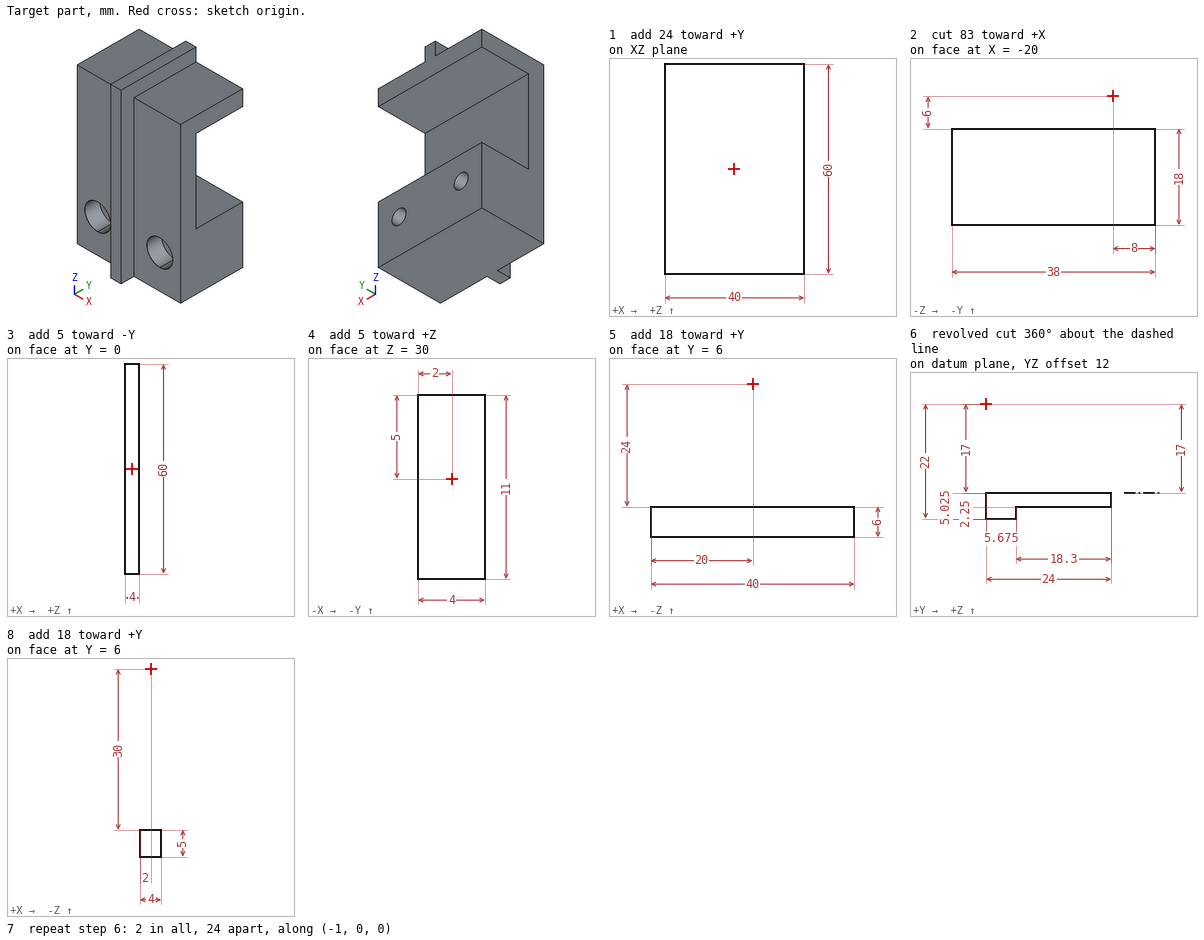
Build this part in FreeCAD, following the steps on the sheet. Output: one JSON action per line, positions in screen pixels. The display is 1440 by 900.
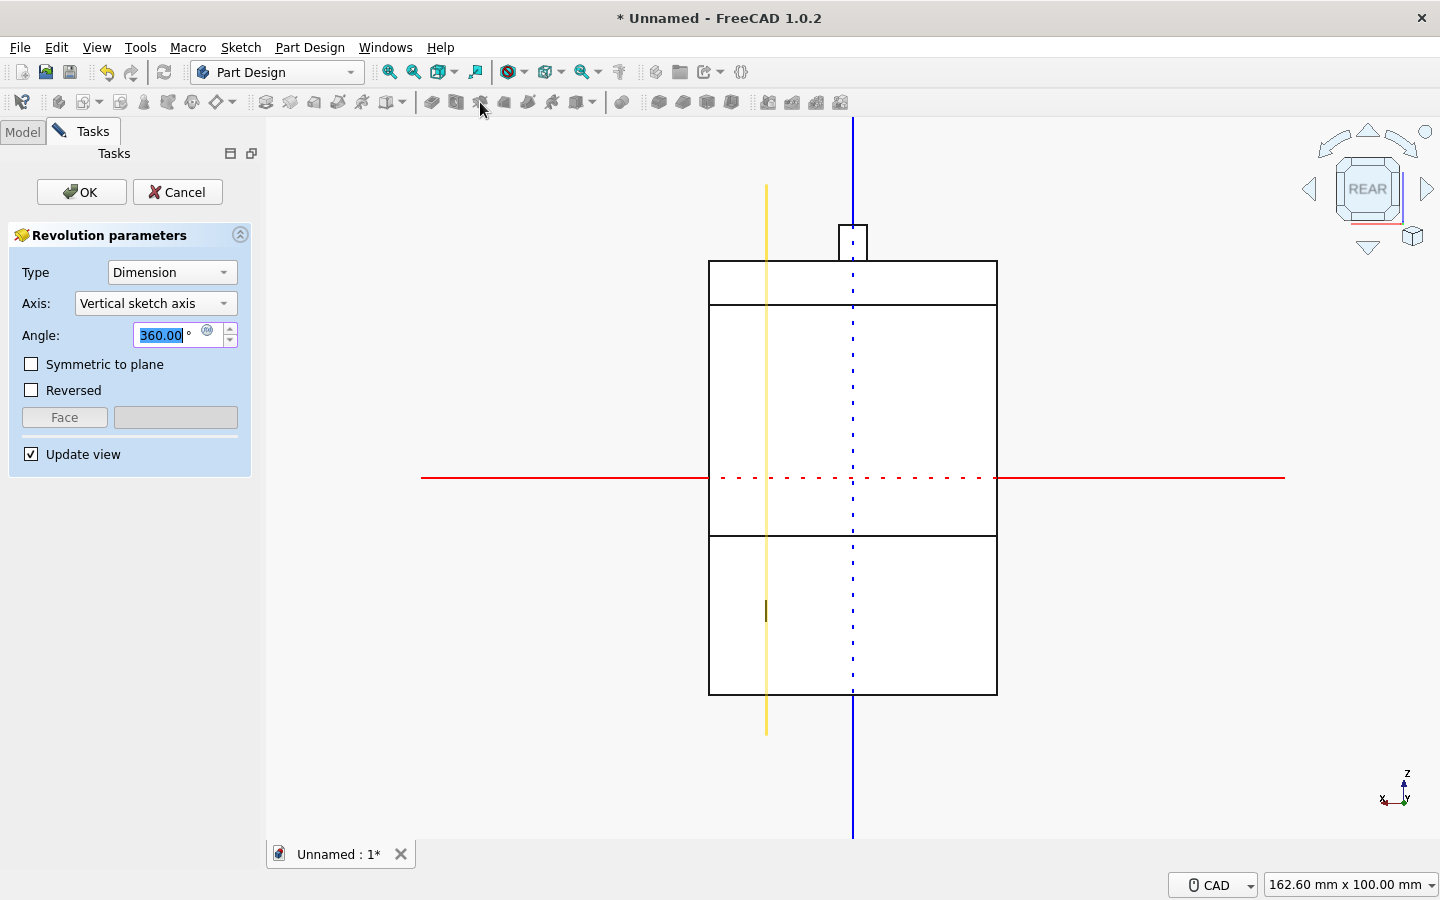
{"action": "left_click", "coordinate": [156, 304]}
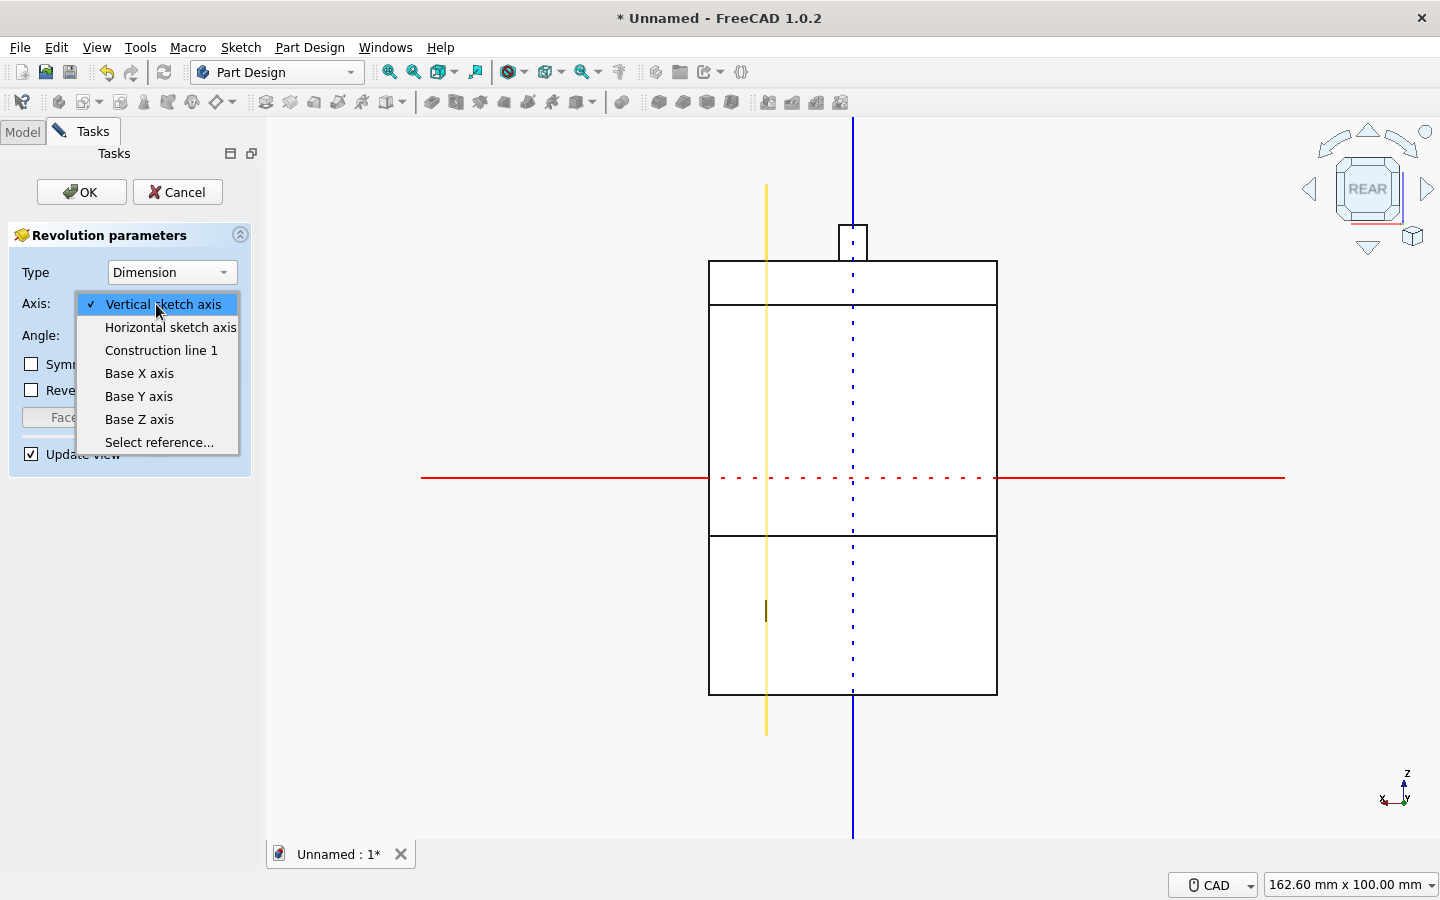
{"action": "left_click", "coordinate": [156, 350]}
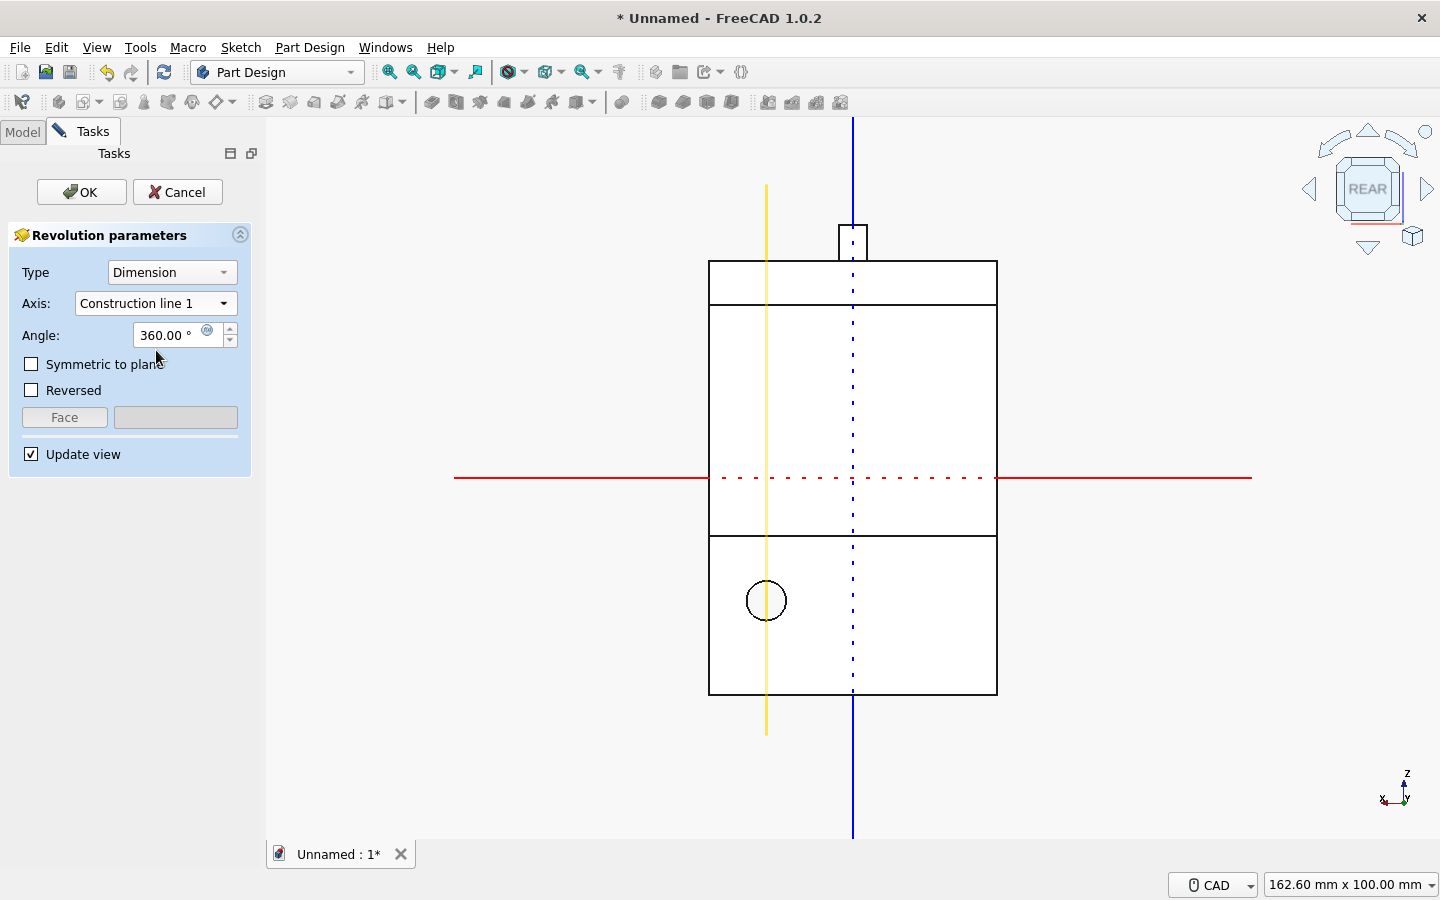
{"action": "left_click", "coordinate": [82, 192]}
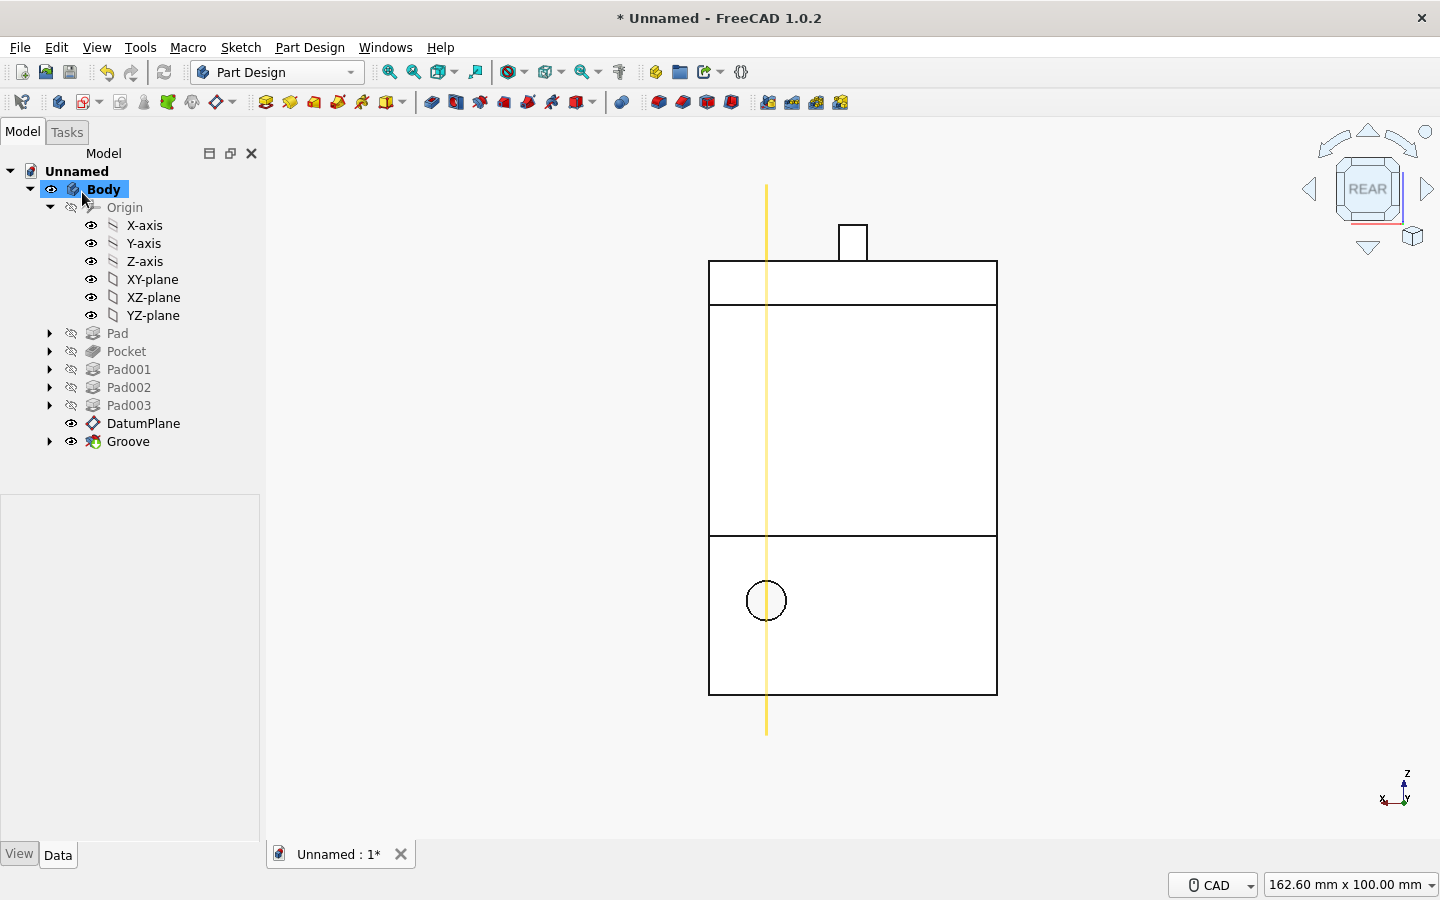
{"action": "left_click", "coordinate": [116, 423]}
{"action": "key", "text": "space"}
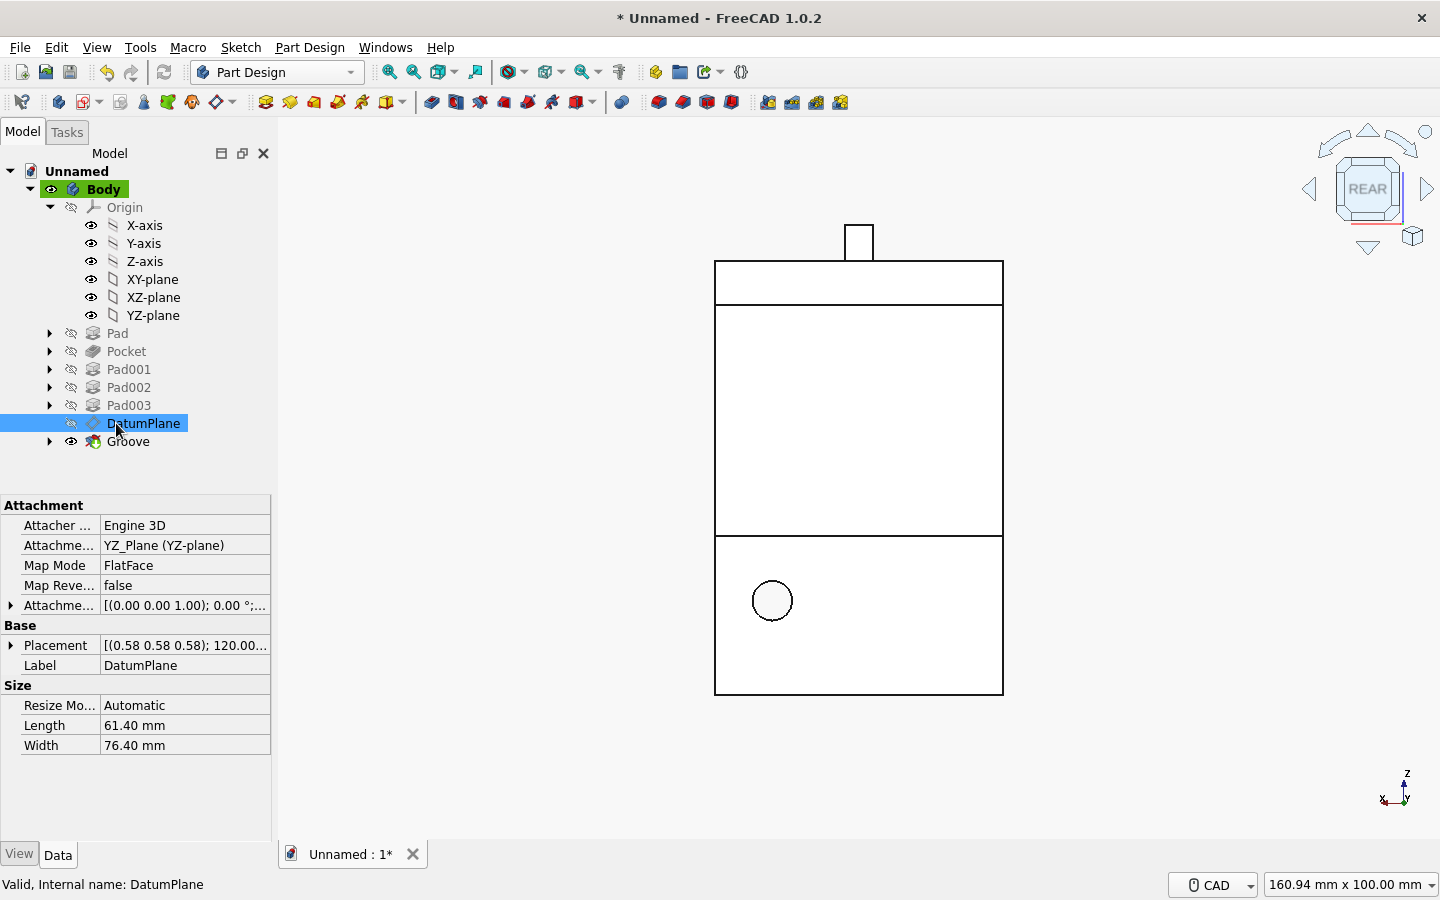
{"action": "left_click", "coordinate": [116, 441]}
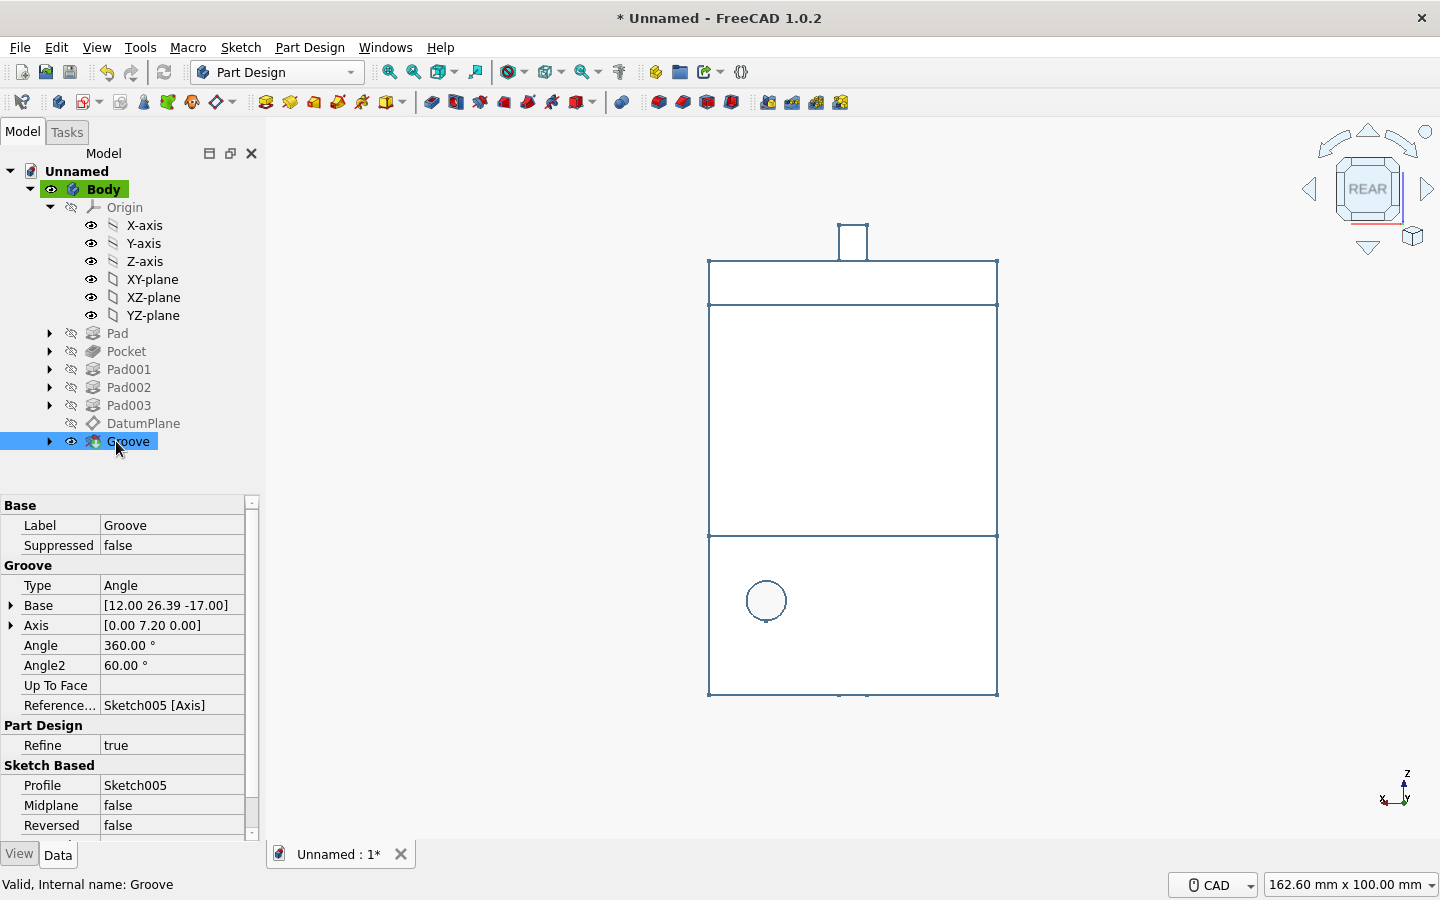
{"action": "left_click", "coordinate": [792, 102]}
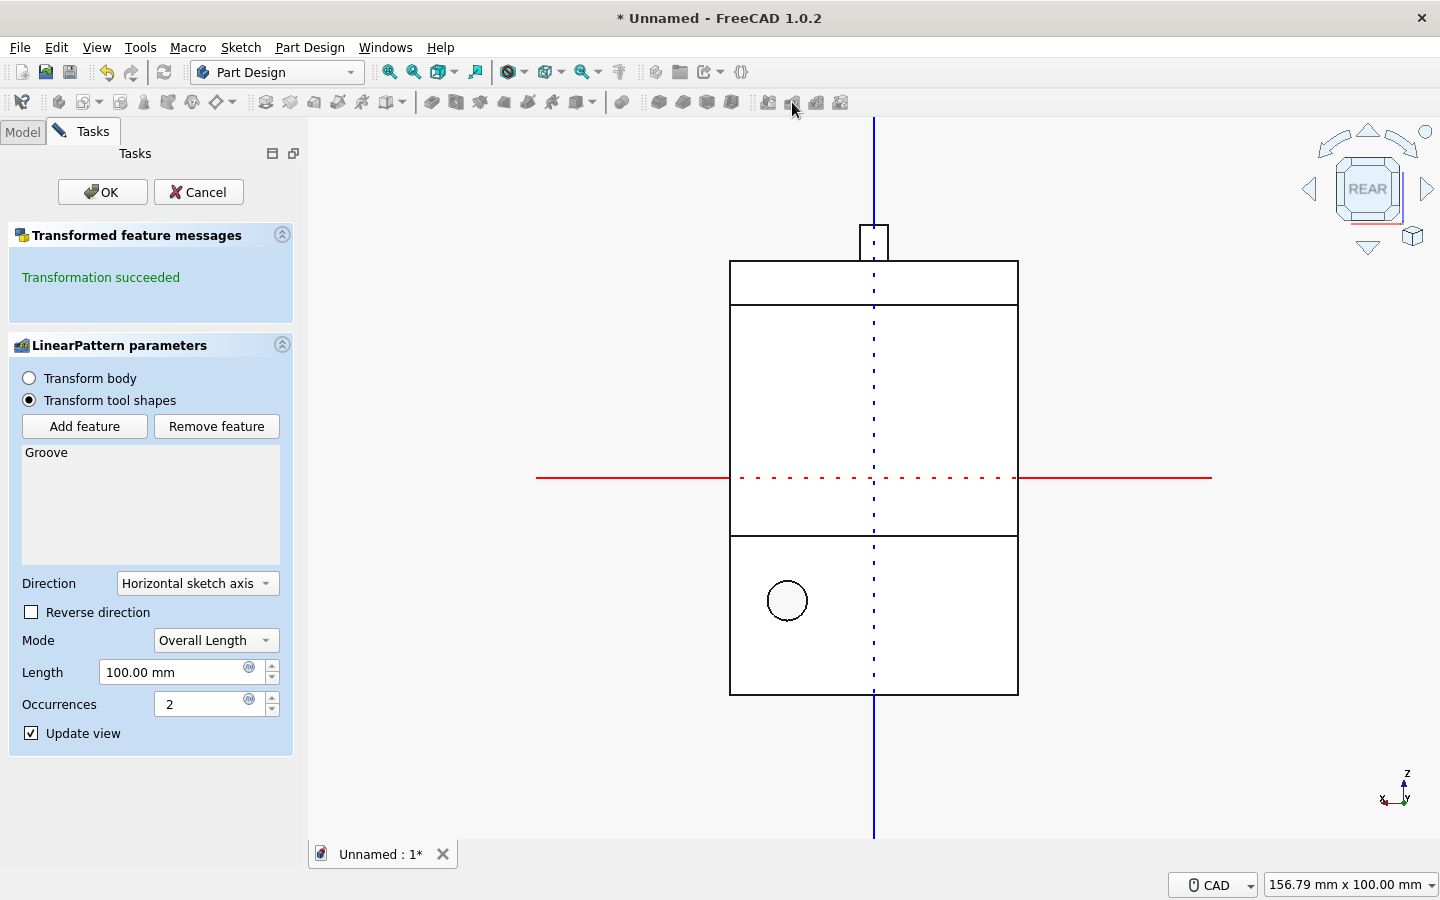
{"action": "left_click", "coordinate": [198, 584]}